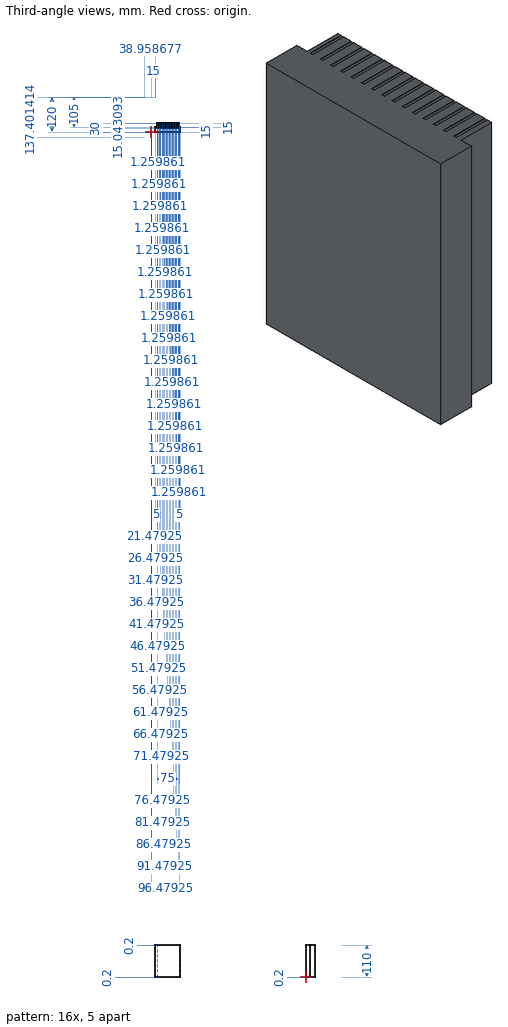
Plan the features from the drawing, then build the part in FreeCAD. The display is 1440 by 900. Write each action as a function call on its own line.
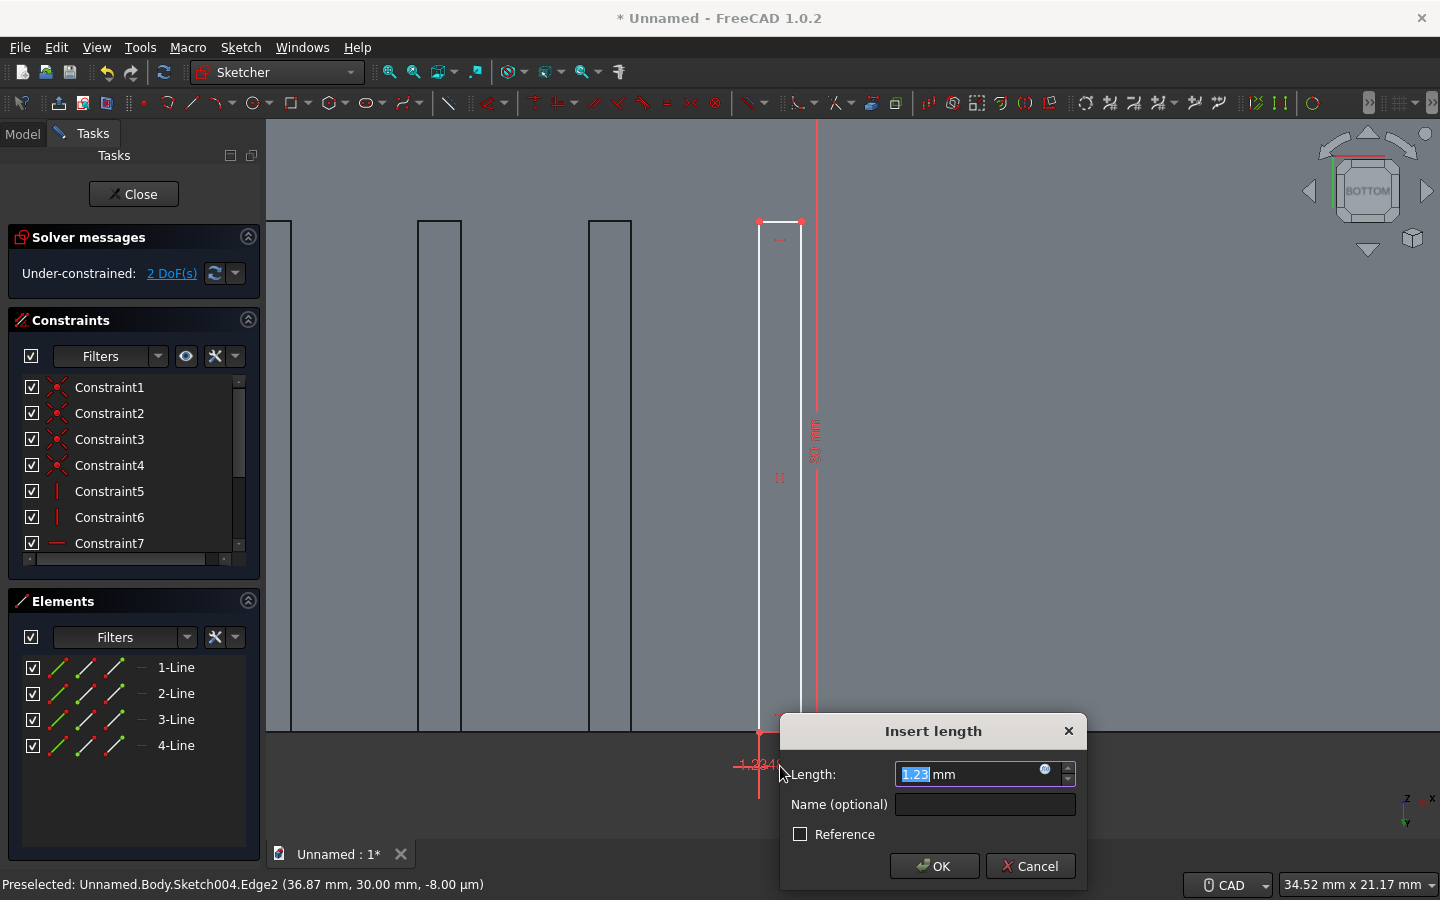
text(1.259861)
key(Return)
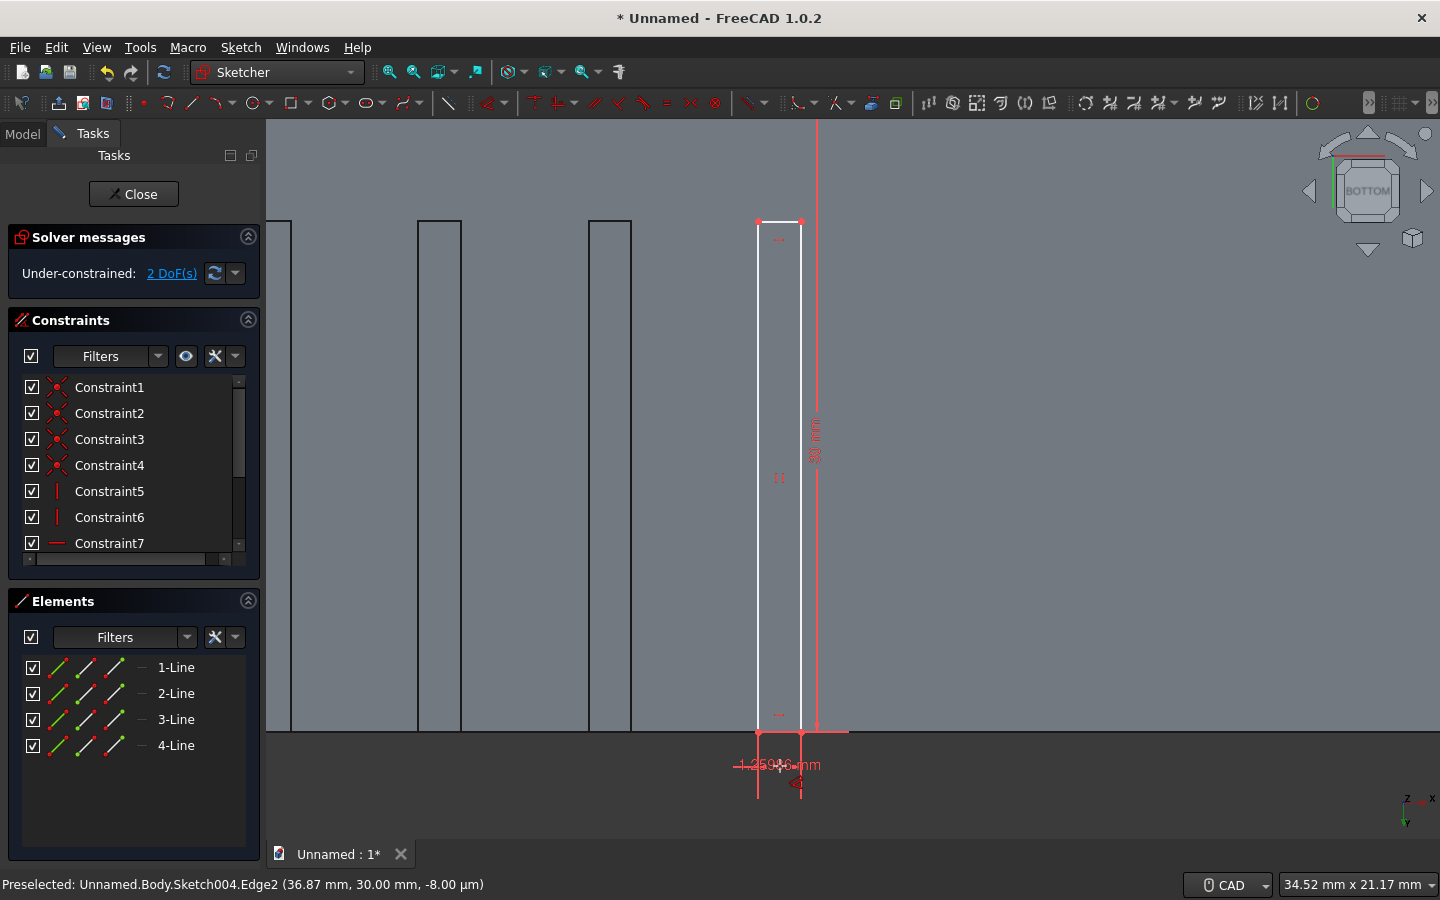
click(758, 375)
click(724, 477)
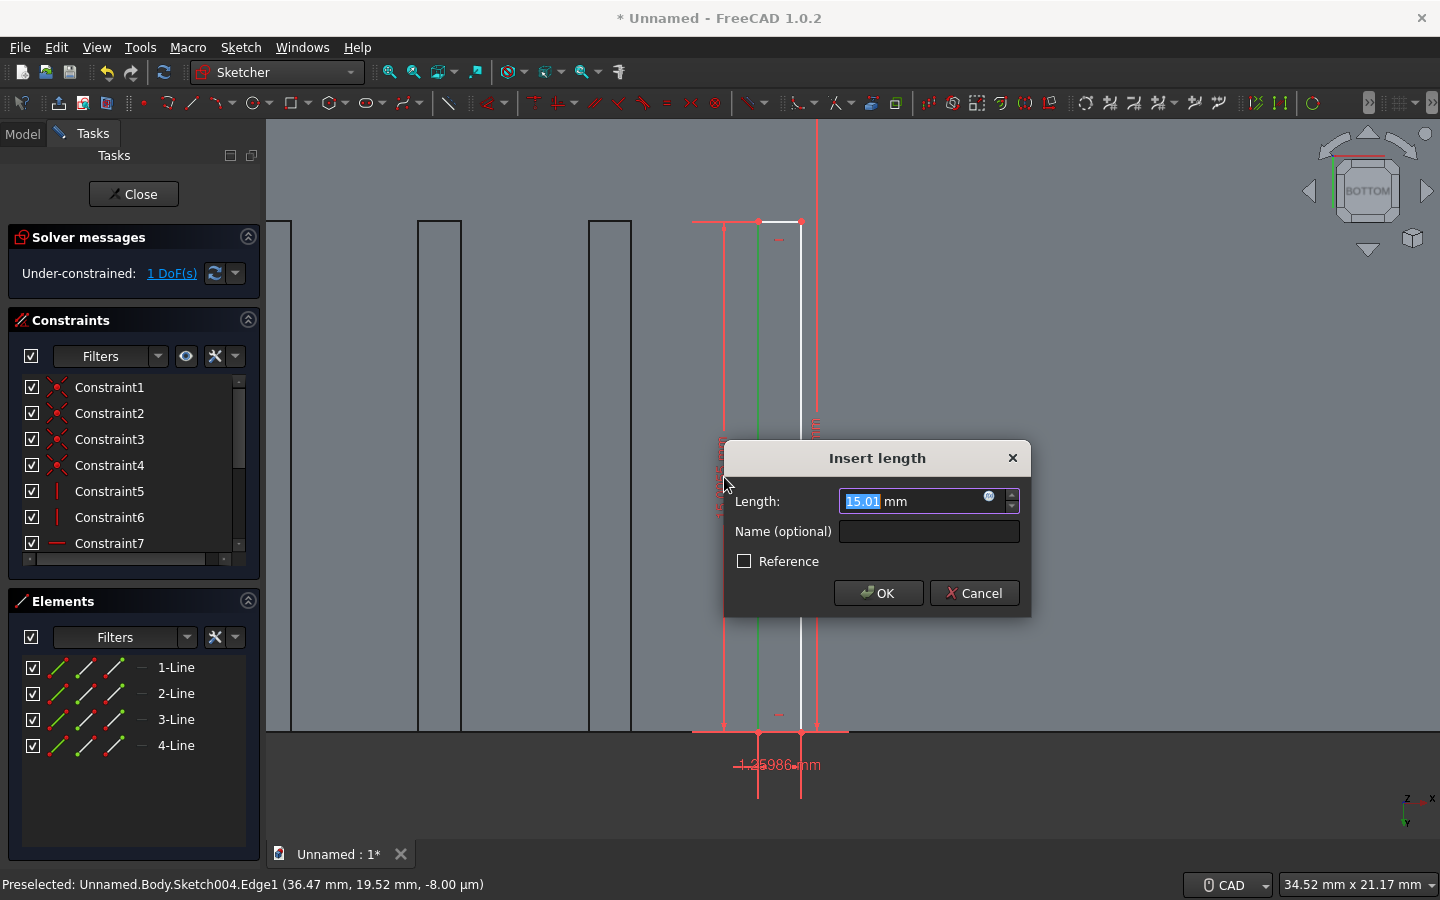
text(15.043093)
key(Return)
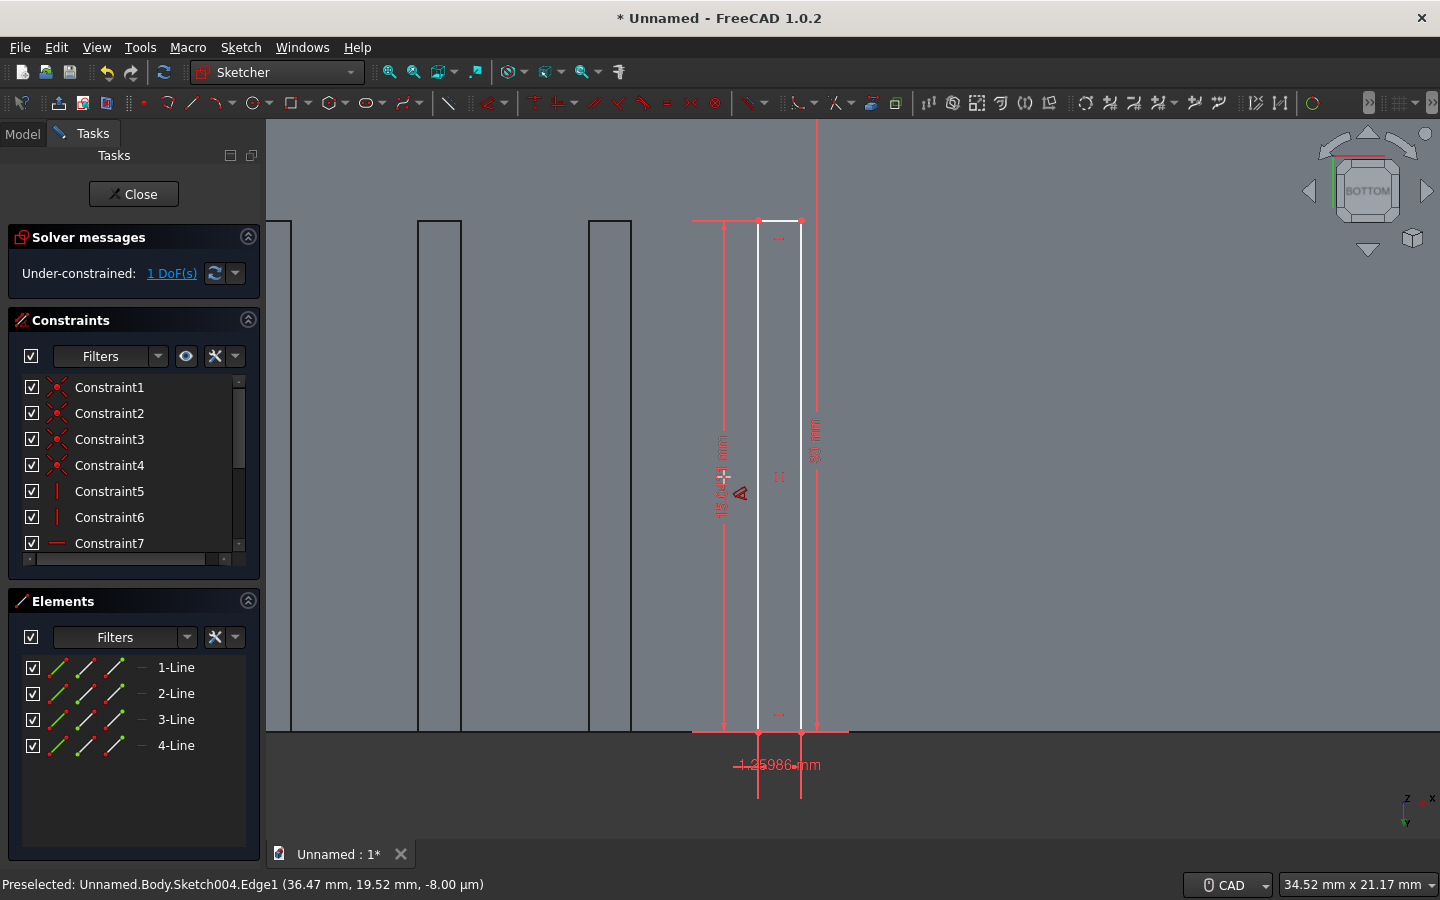
click(758, 221)
click(526, 255)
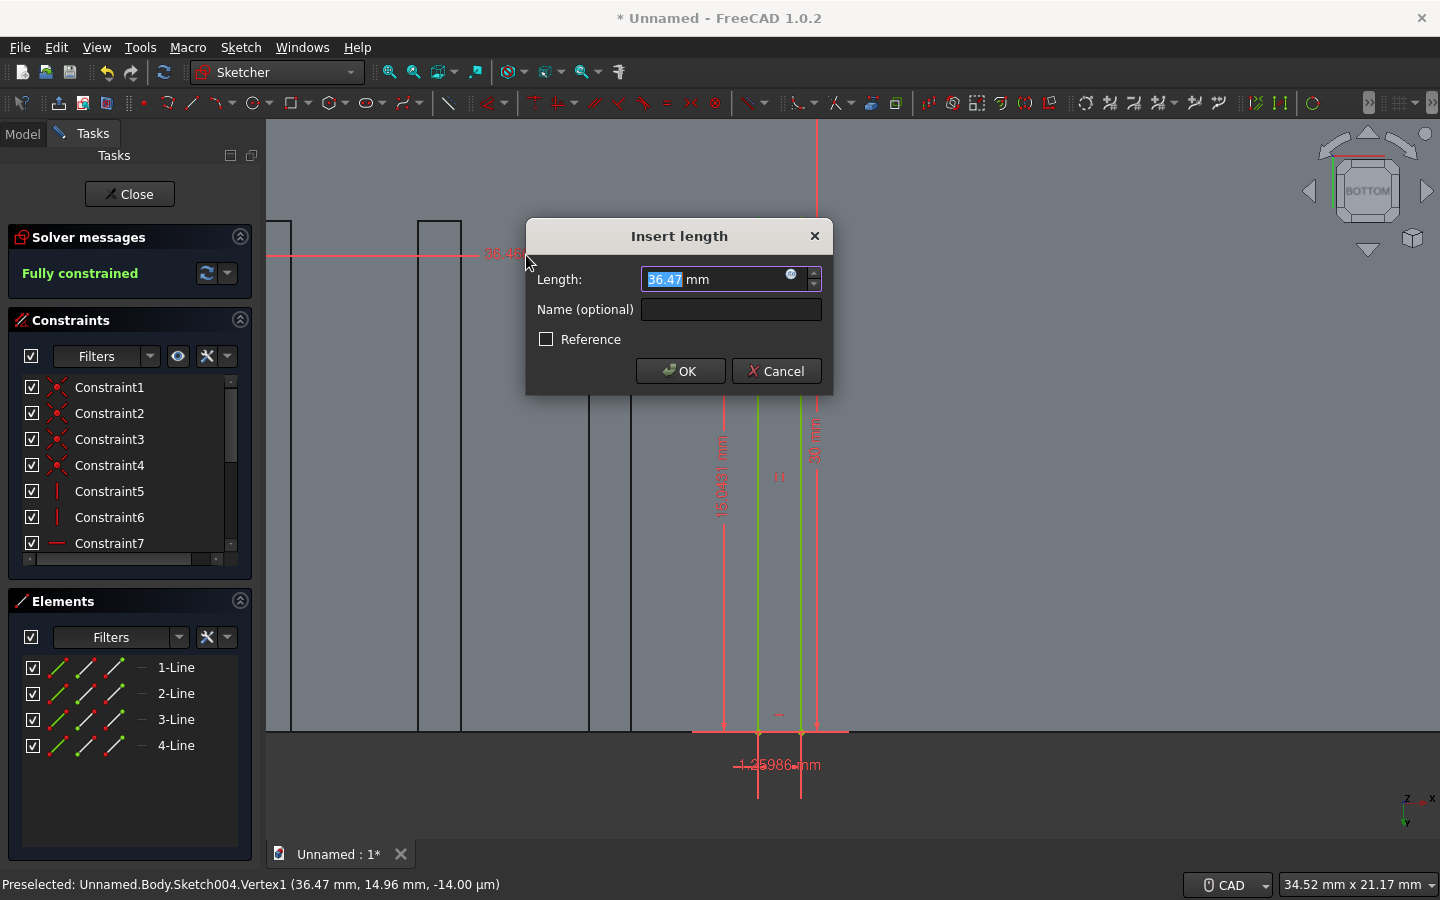
text(36.47925)
key(Return)
key(Escape)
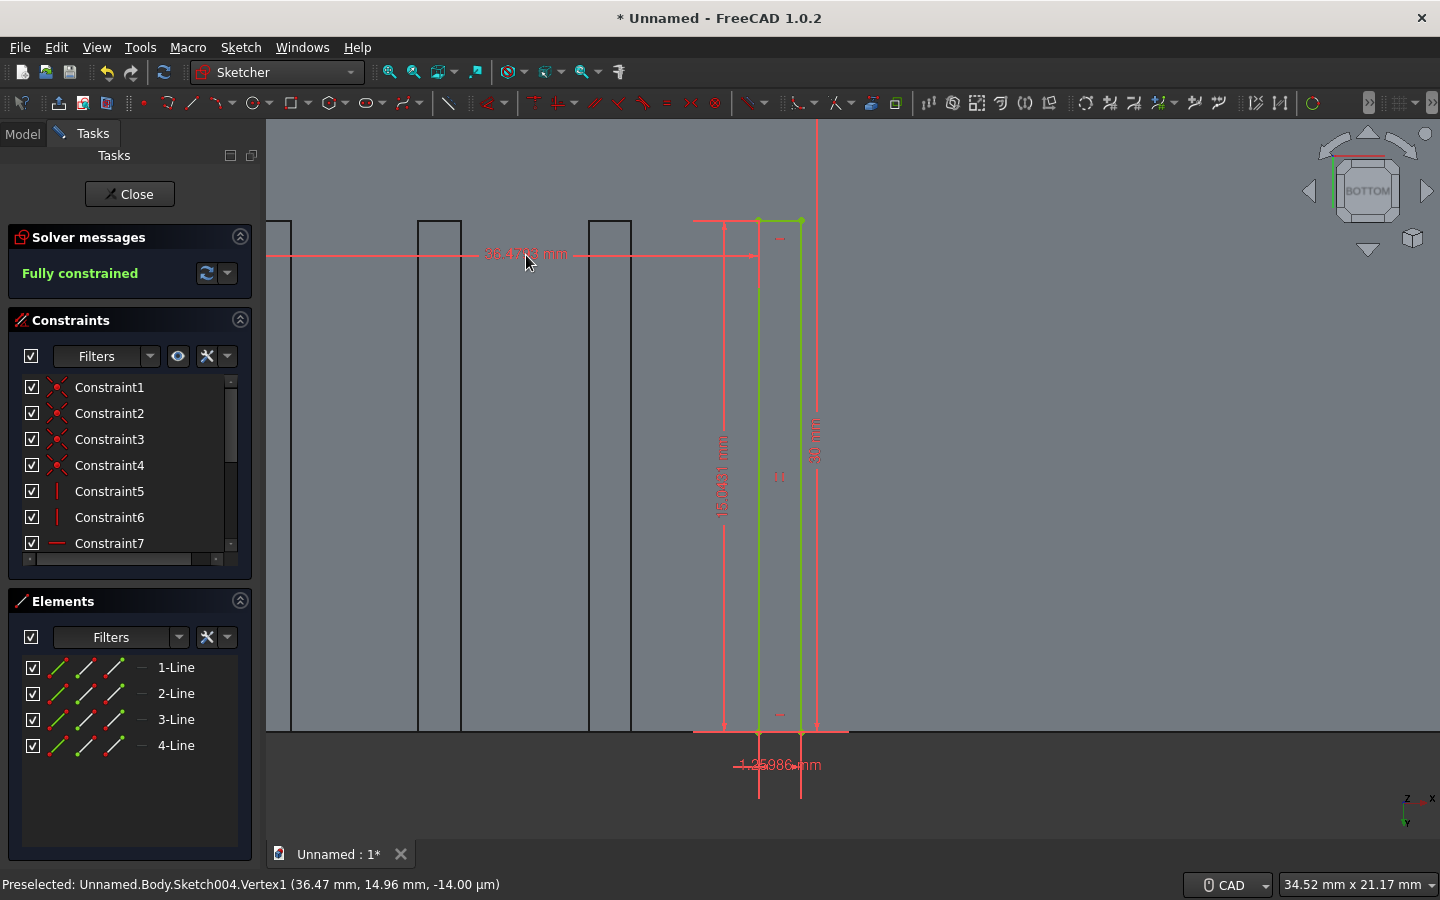
click(130, 194)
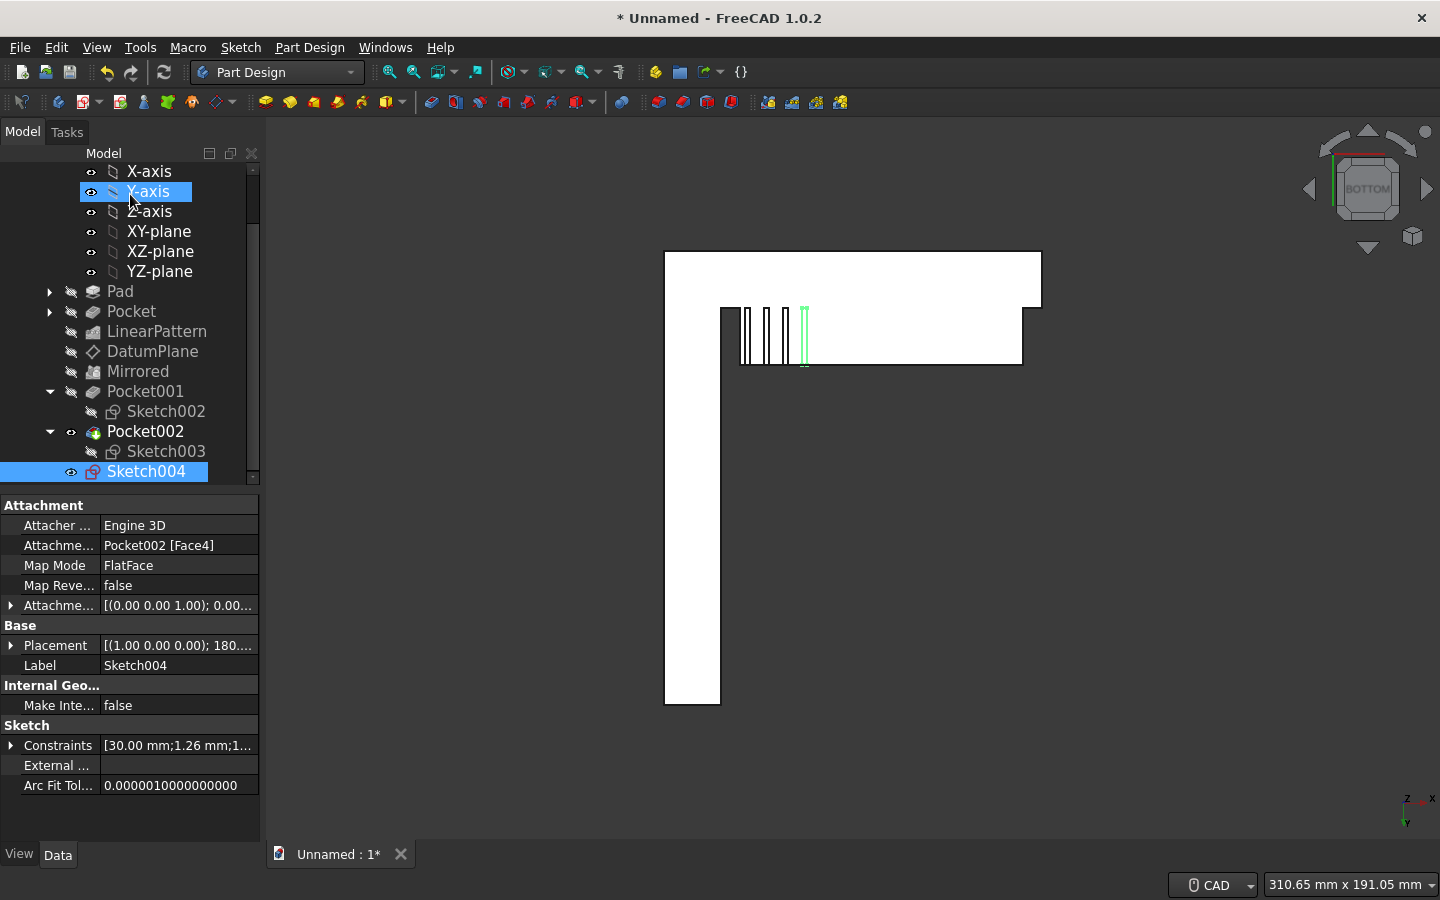
click(432, 102)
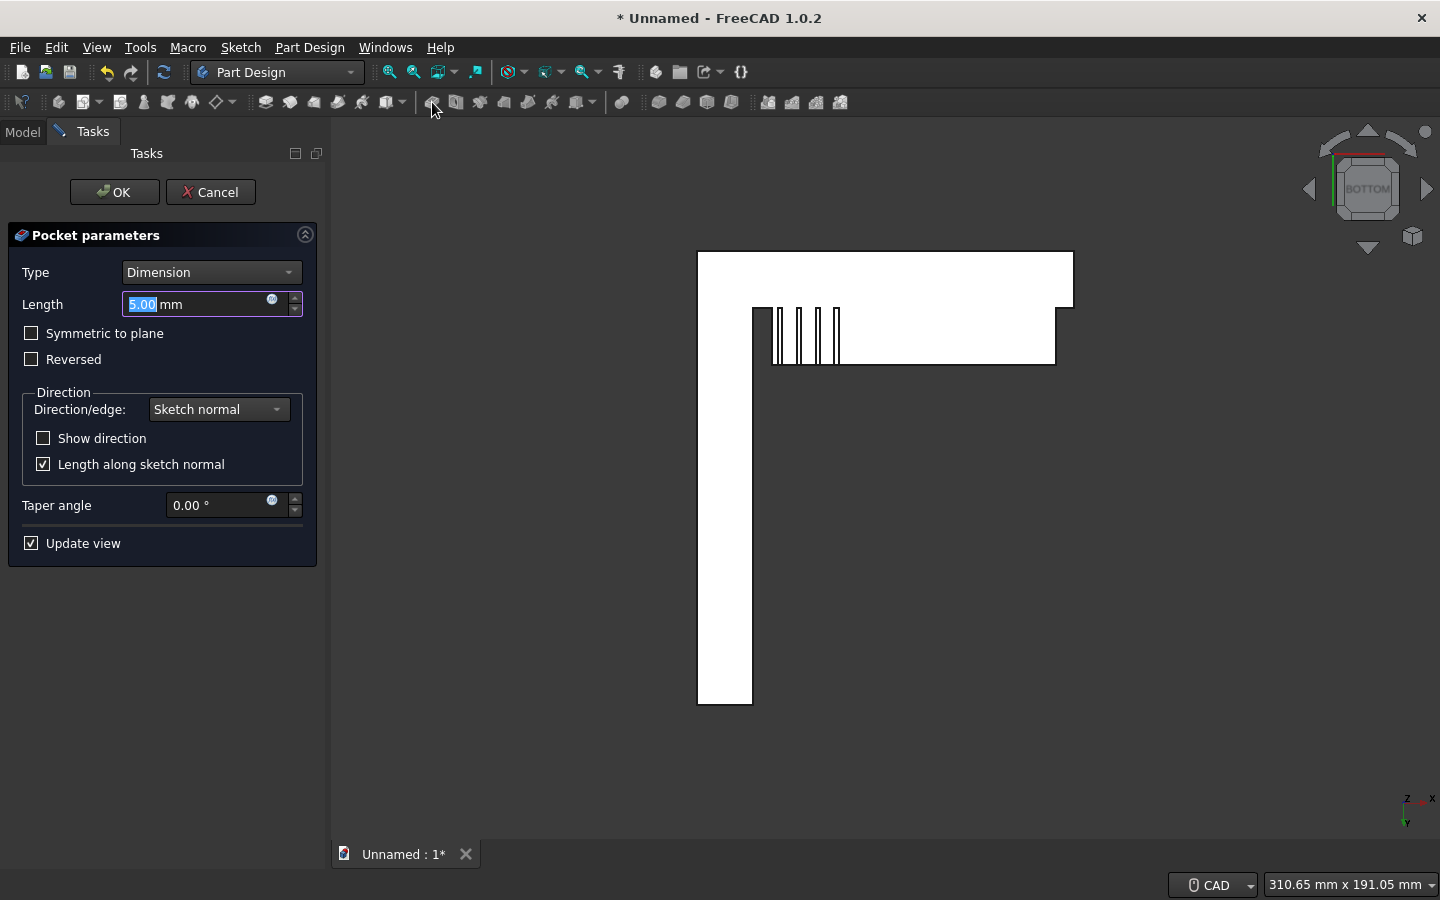
text(0.2)
key(Tab)